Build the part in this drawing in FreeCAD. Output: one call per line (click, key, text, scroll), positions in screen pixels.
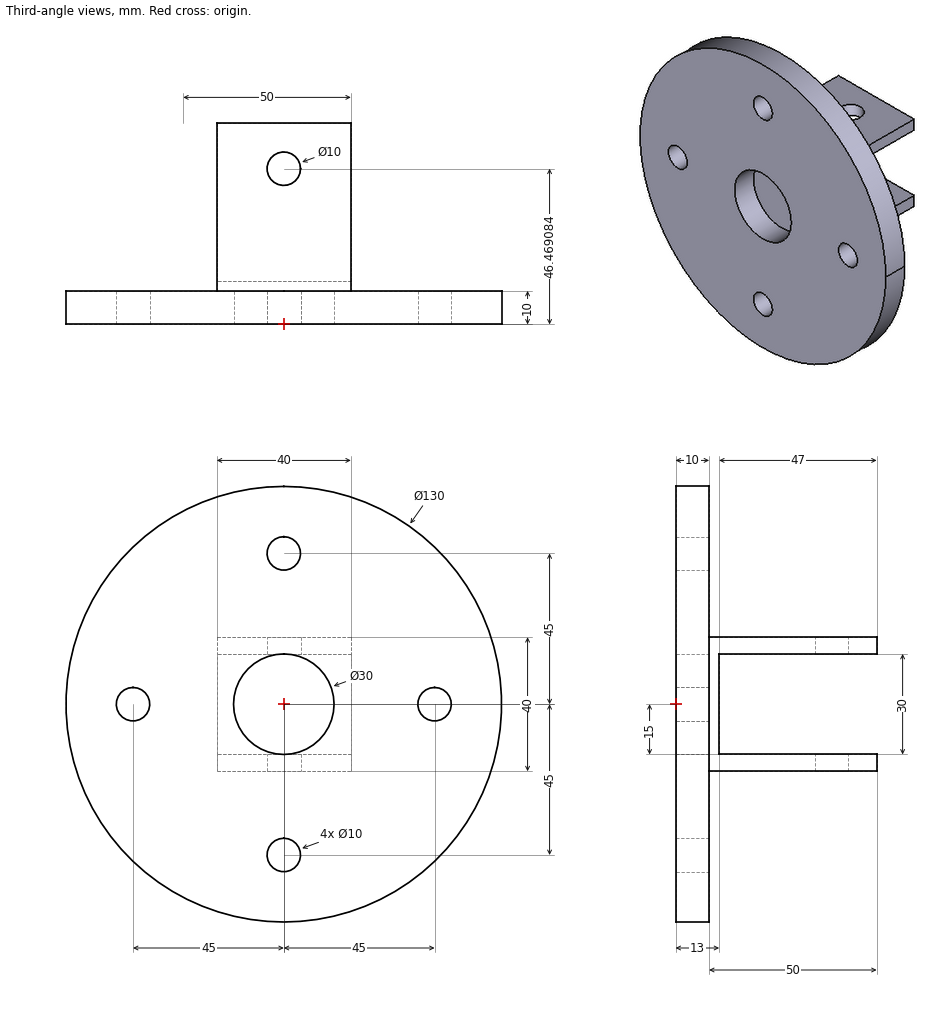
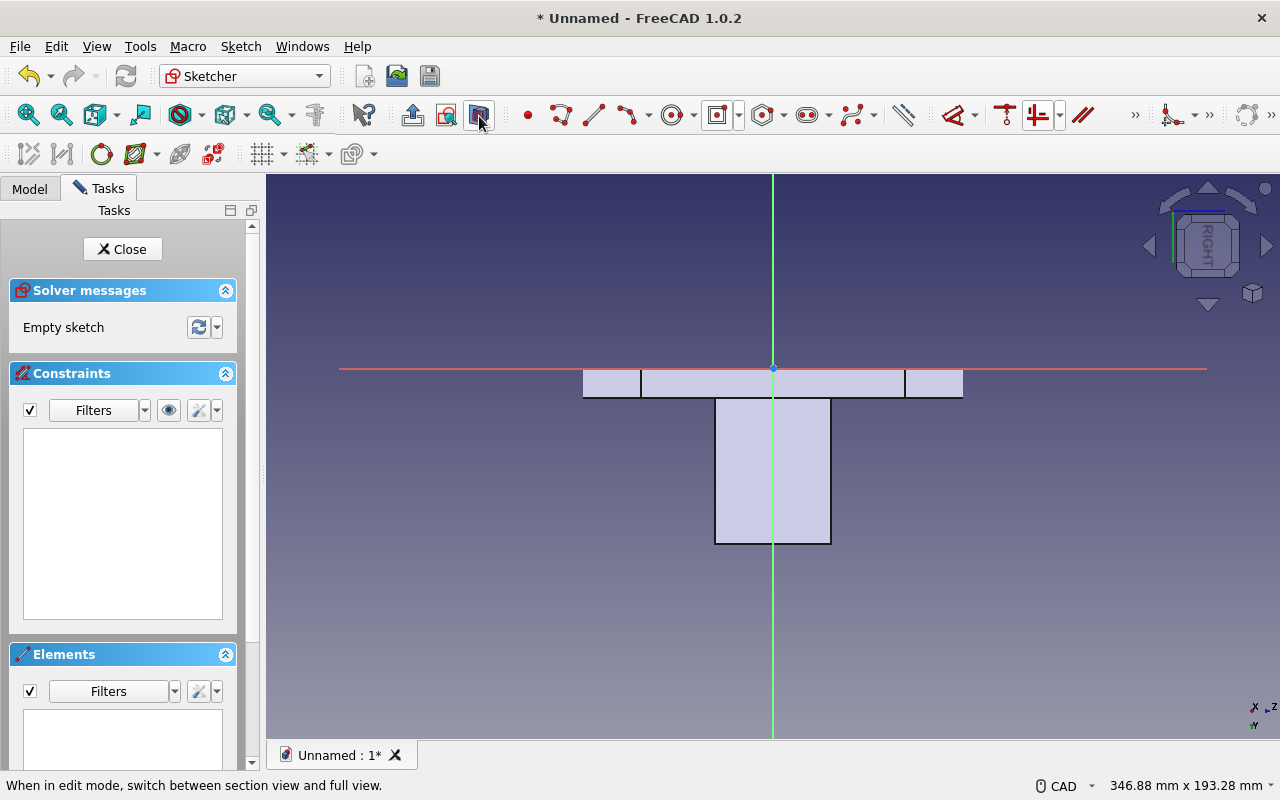
scroll(829, 456, up, 4)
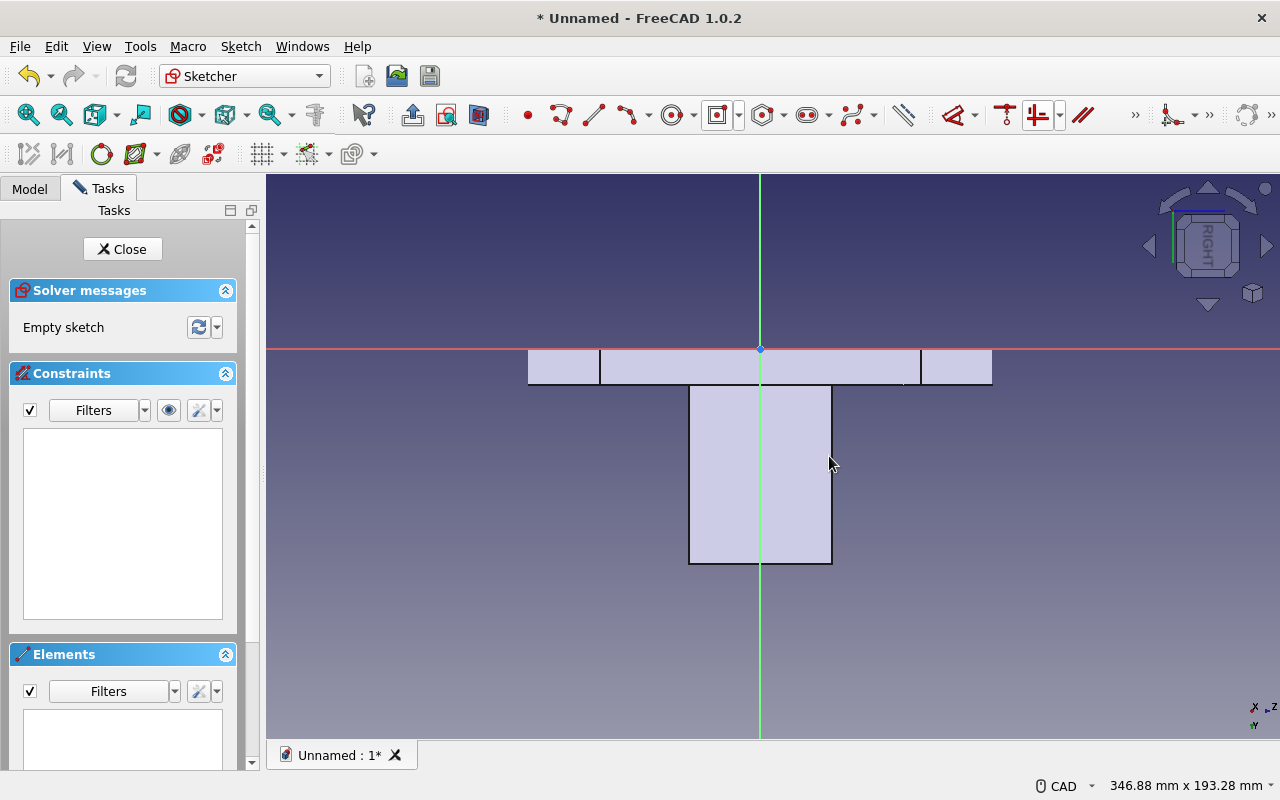
key(g)
key(r)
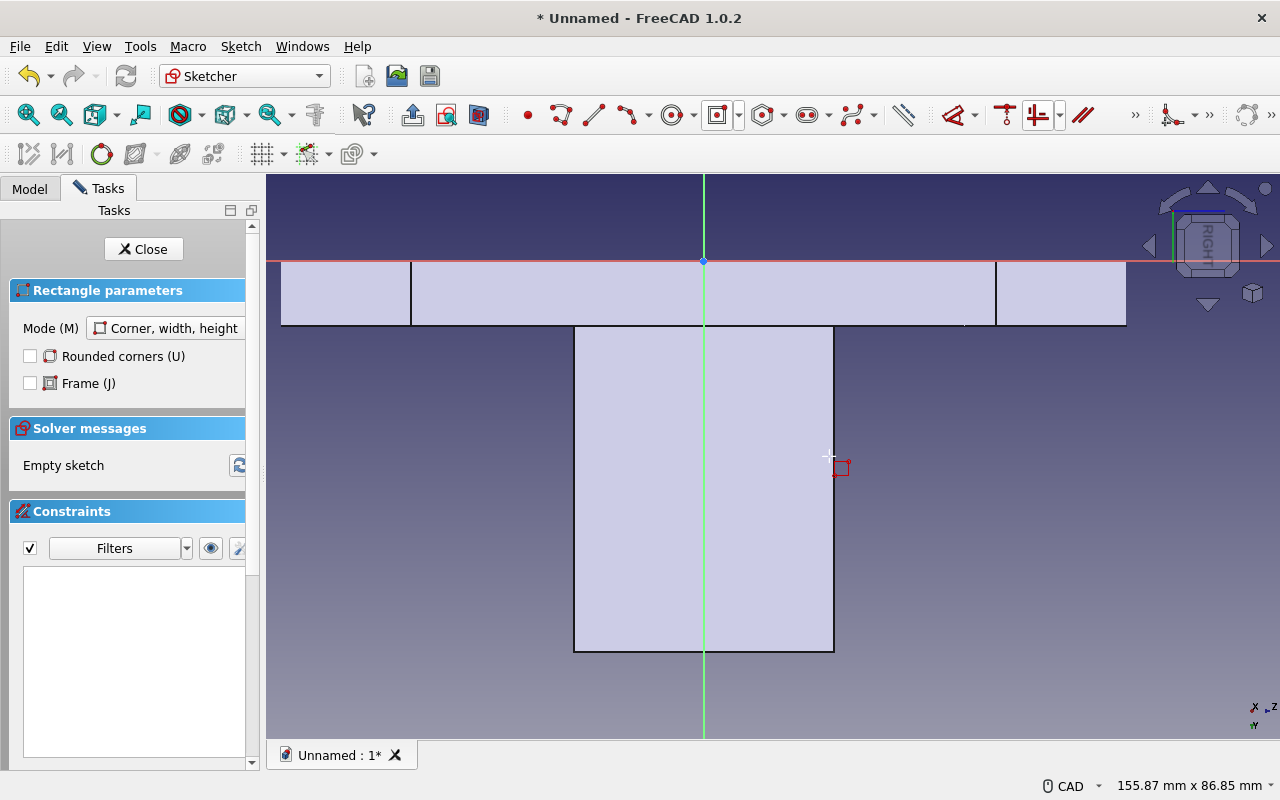
click(606, 346)
move(801, 652)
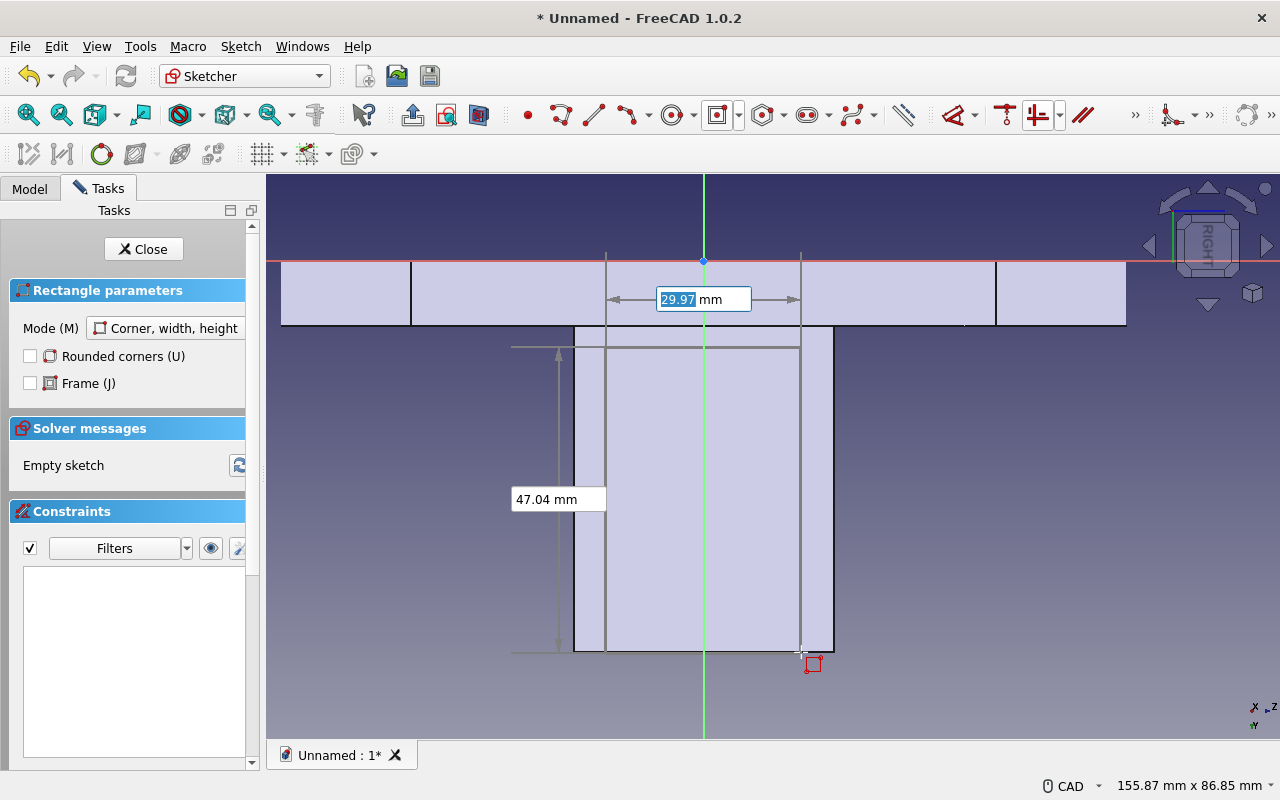
text(30)
key(Tab)
text(47)
key(Return)
key(Escape)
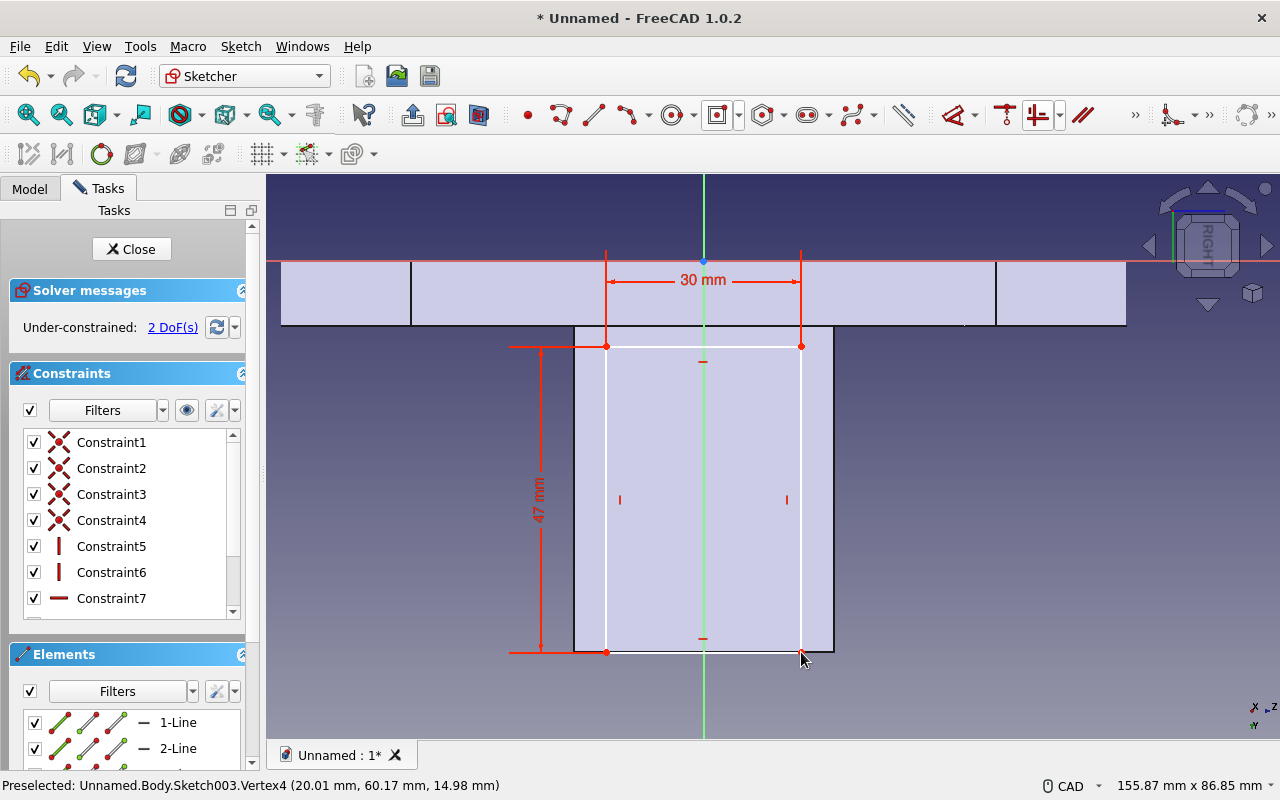
click(952, 116)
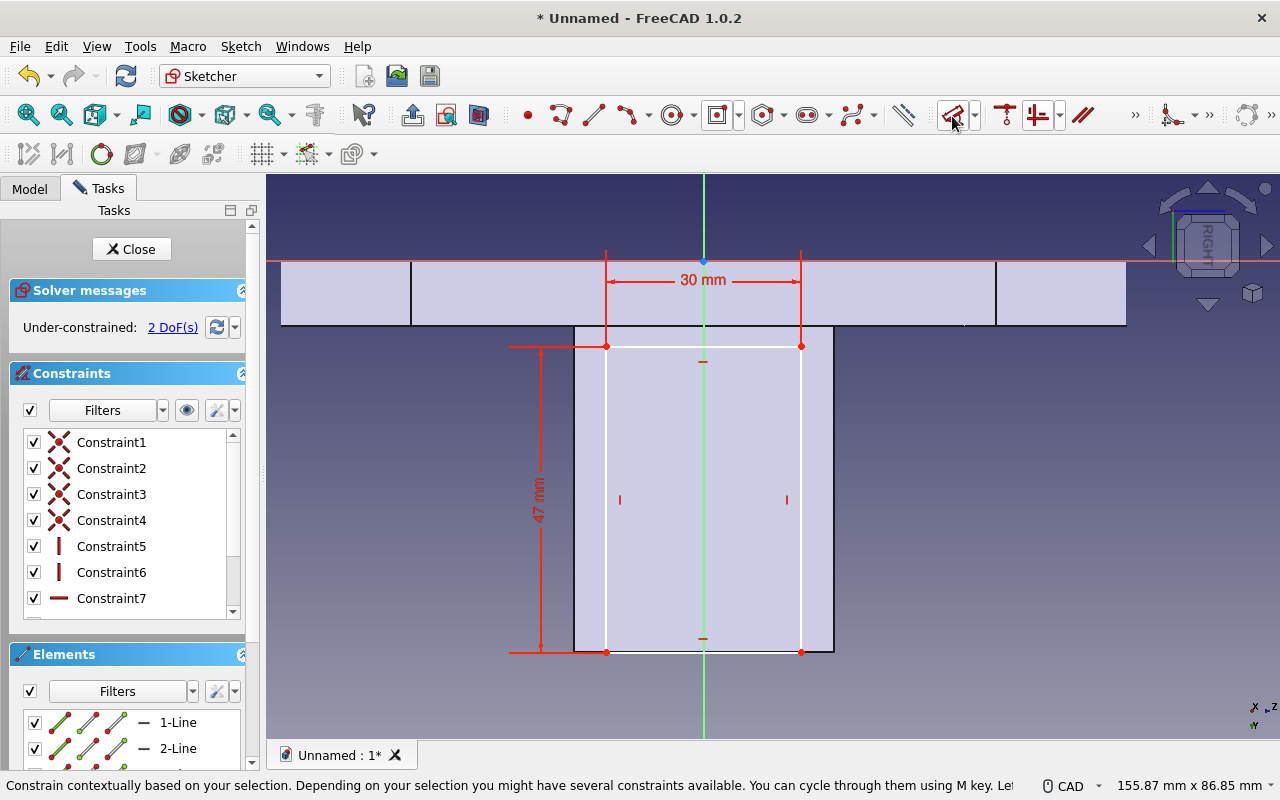
click(606, 347)
click(655, 227)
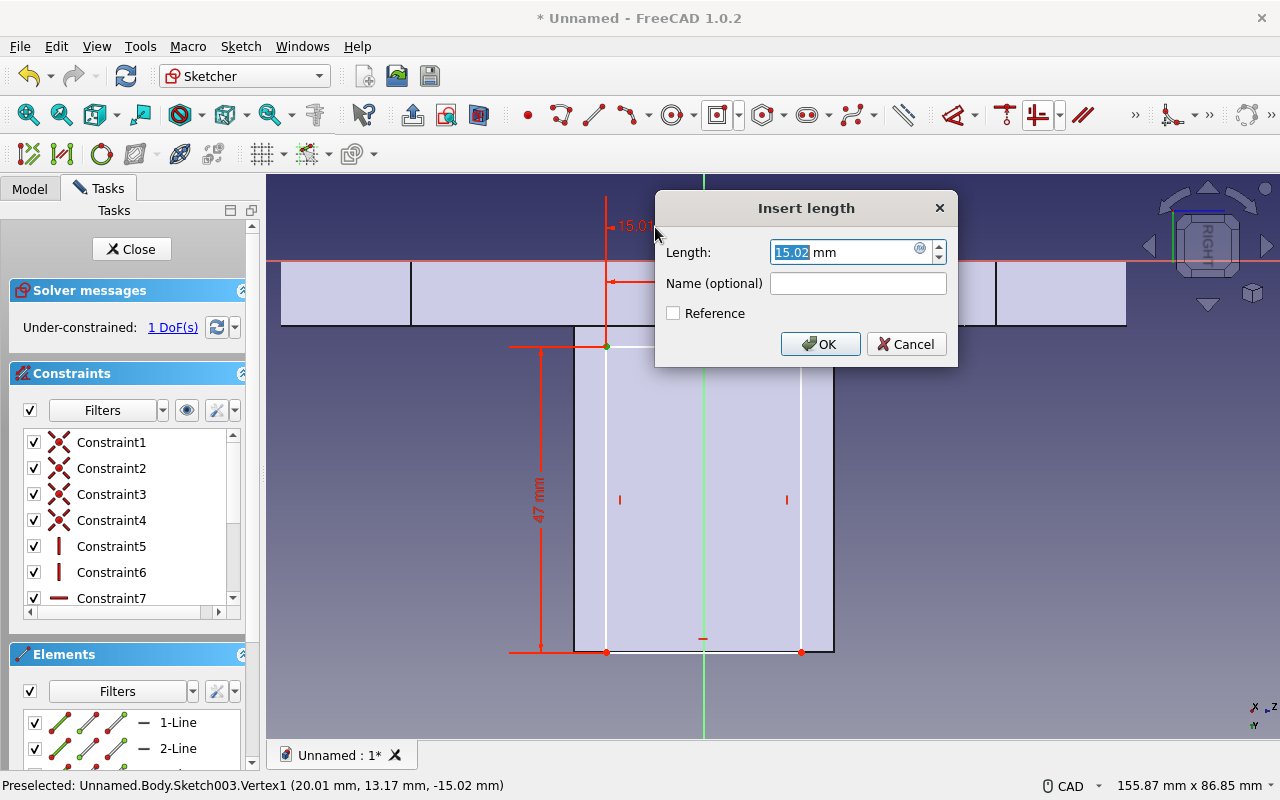
text(15)
key(Return)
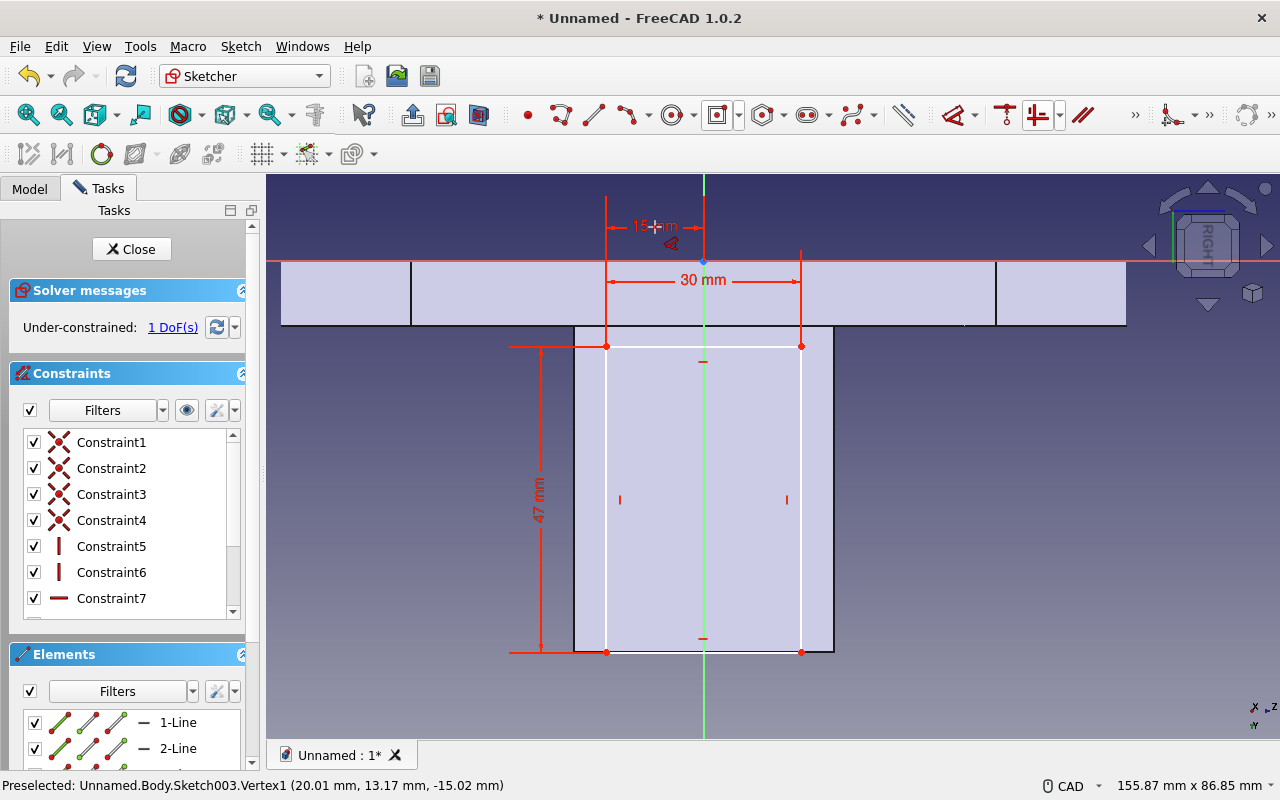
click(606, 347)
click(572, 304)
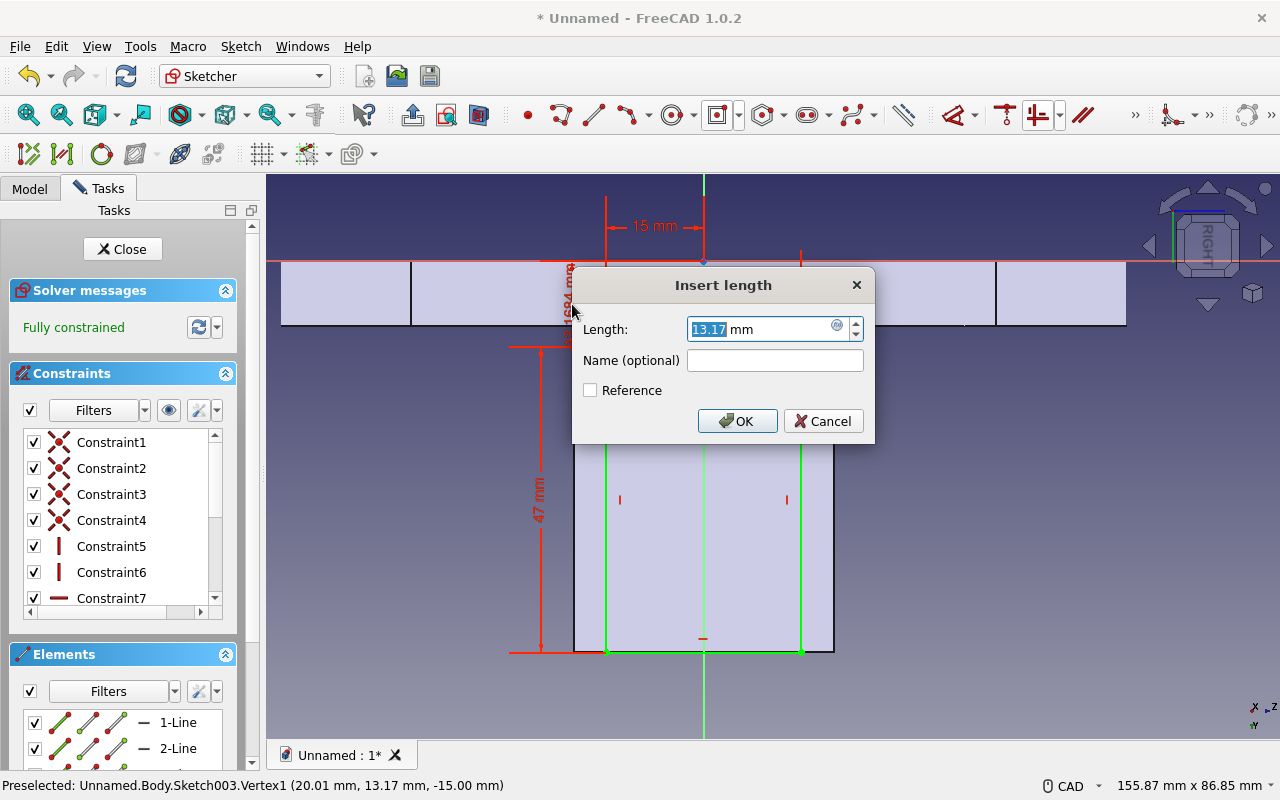
text(13)
key(Return)
key(Escape)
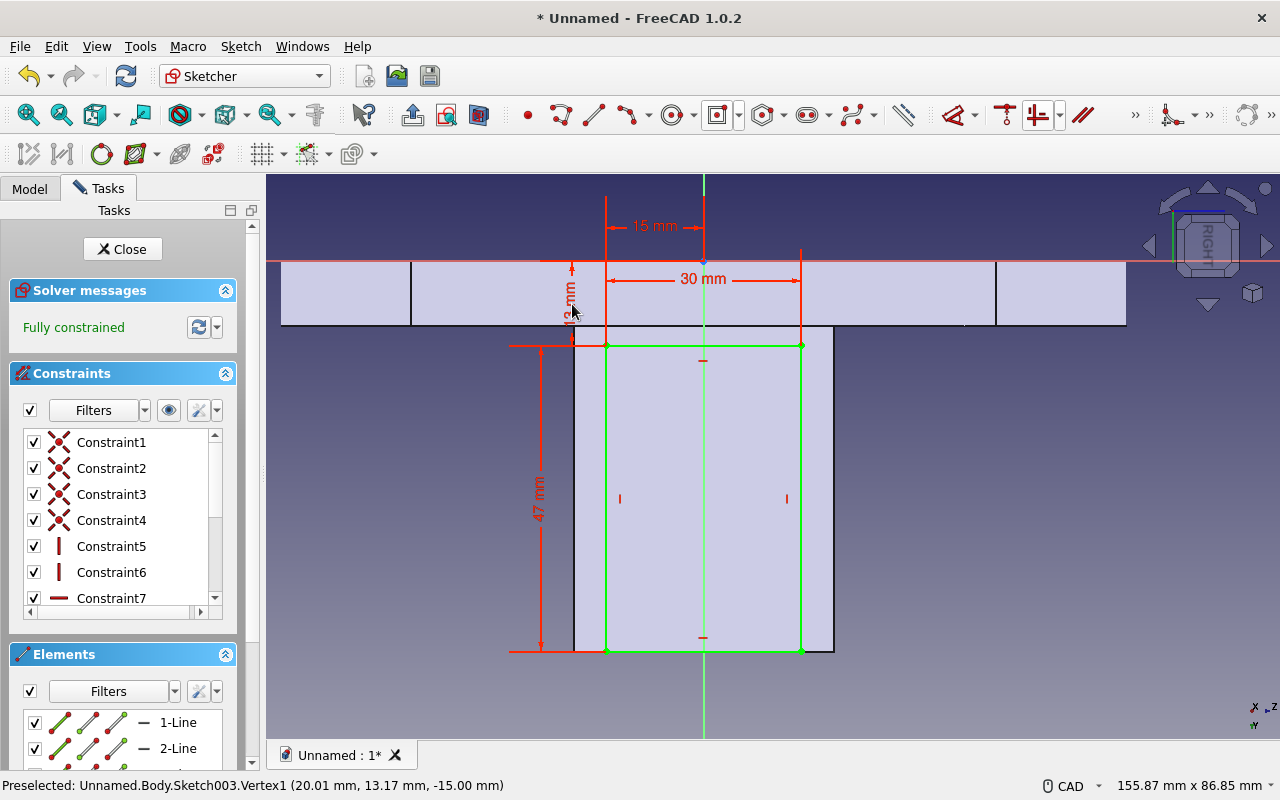
click(123, 249)